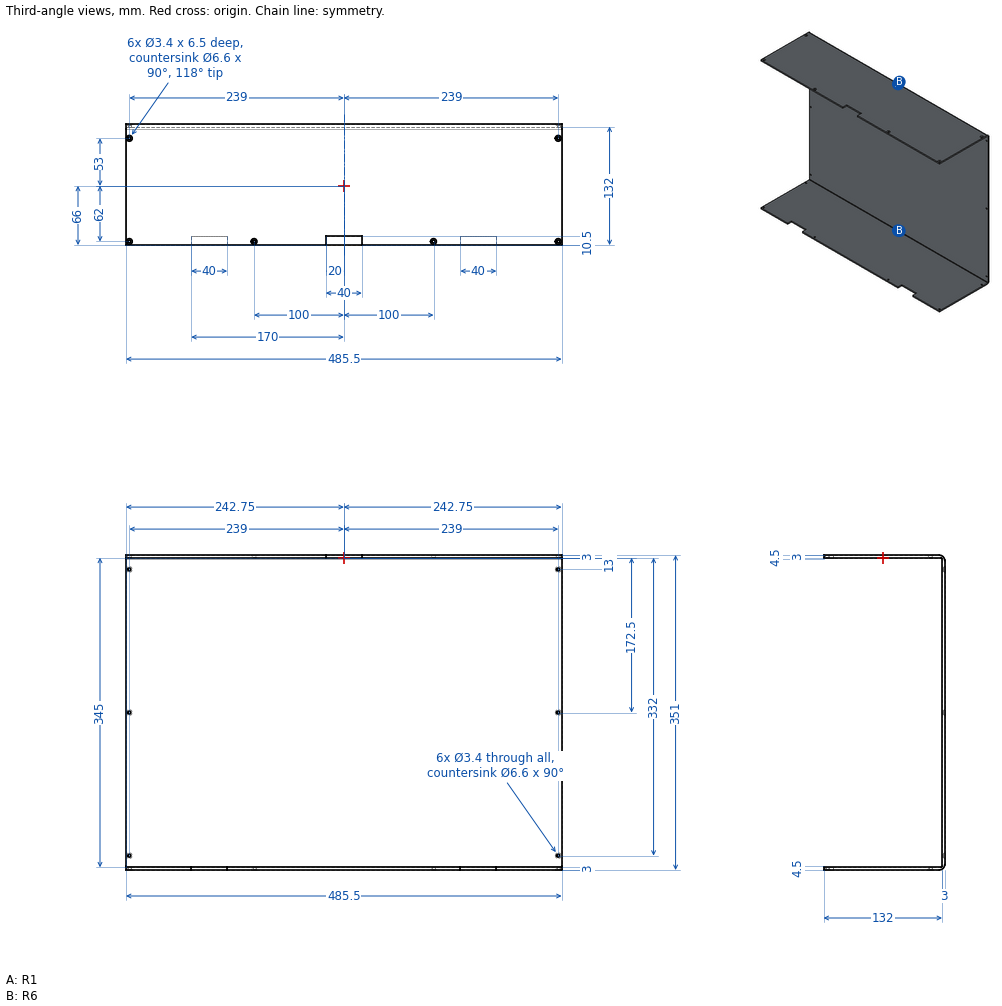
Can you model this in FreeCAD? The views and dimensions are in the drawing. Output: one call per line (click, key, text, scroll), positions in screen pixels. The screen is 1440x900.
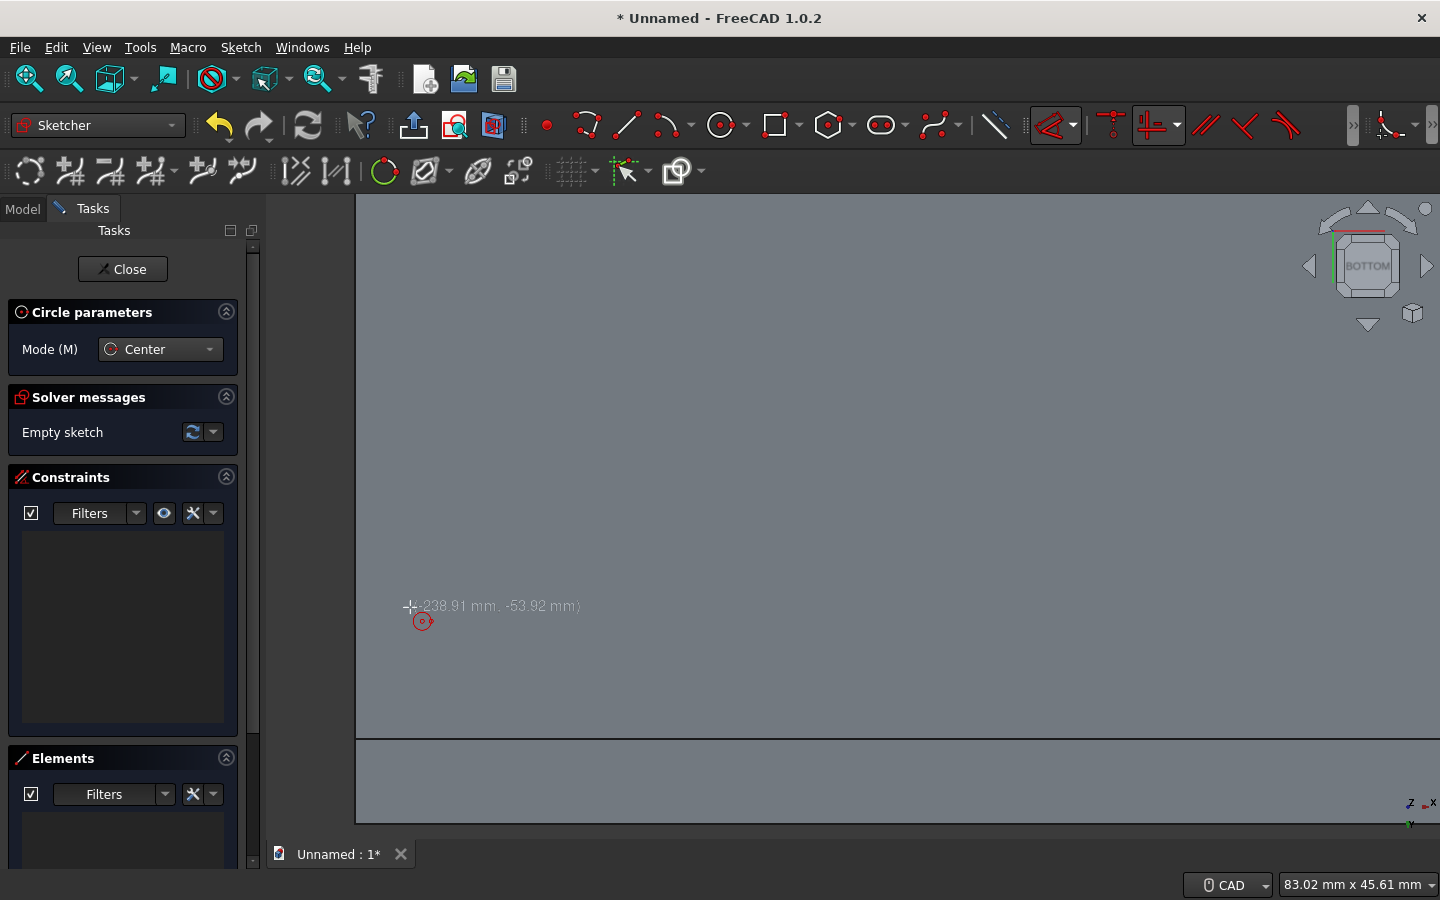
scroll(410, 608, down, 11)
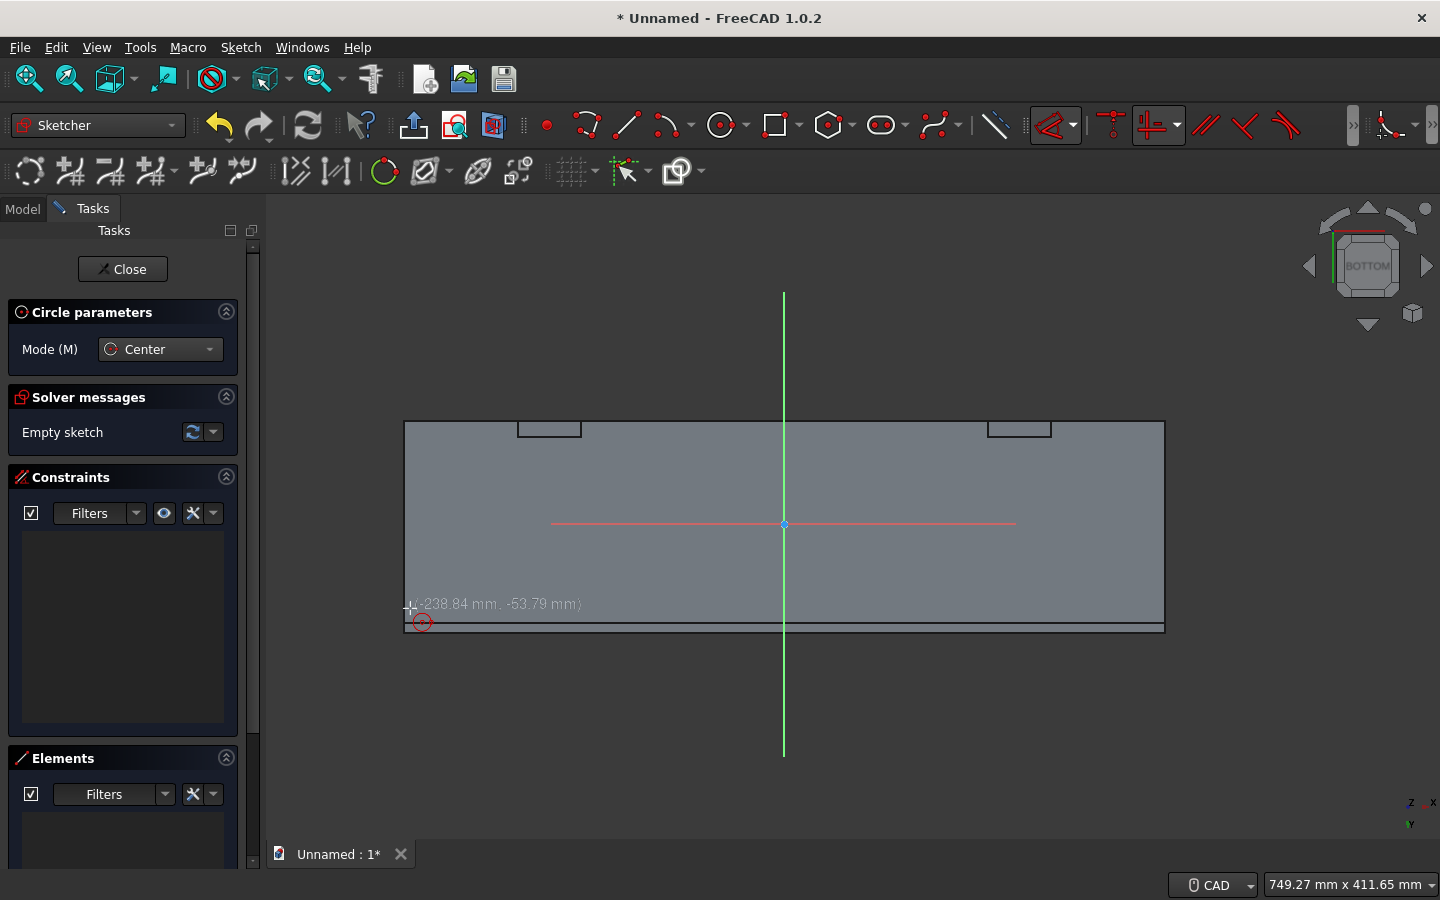
click(410, 607)
move(412, 606)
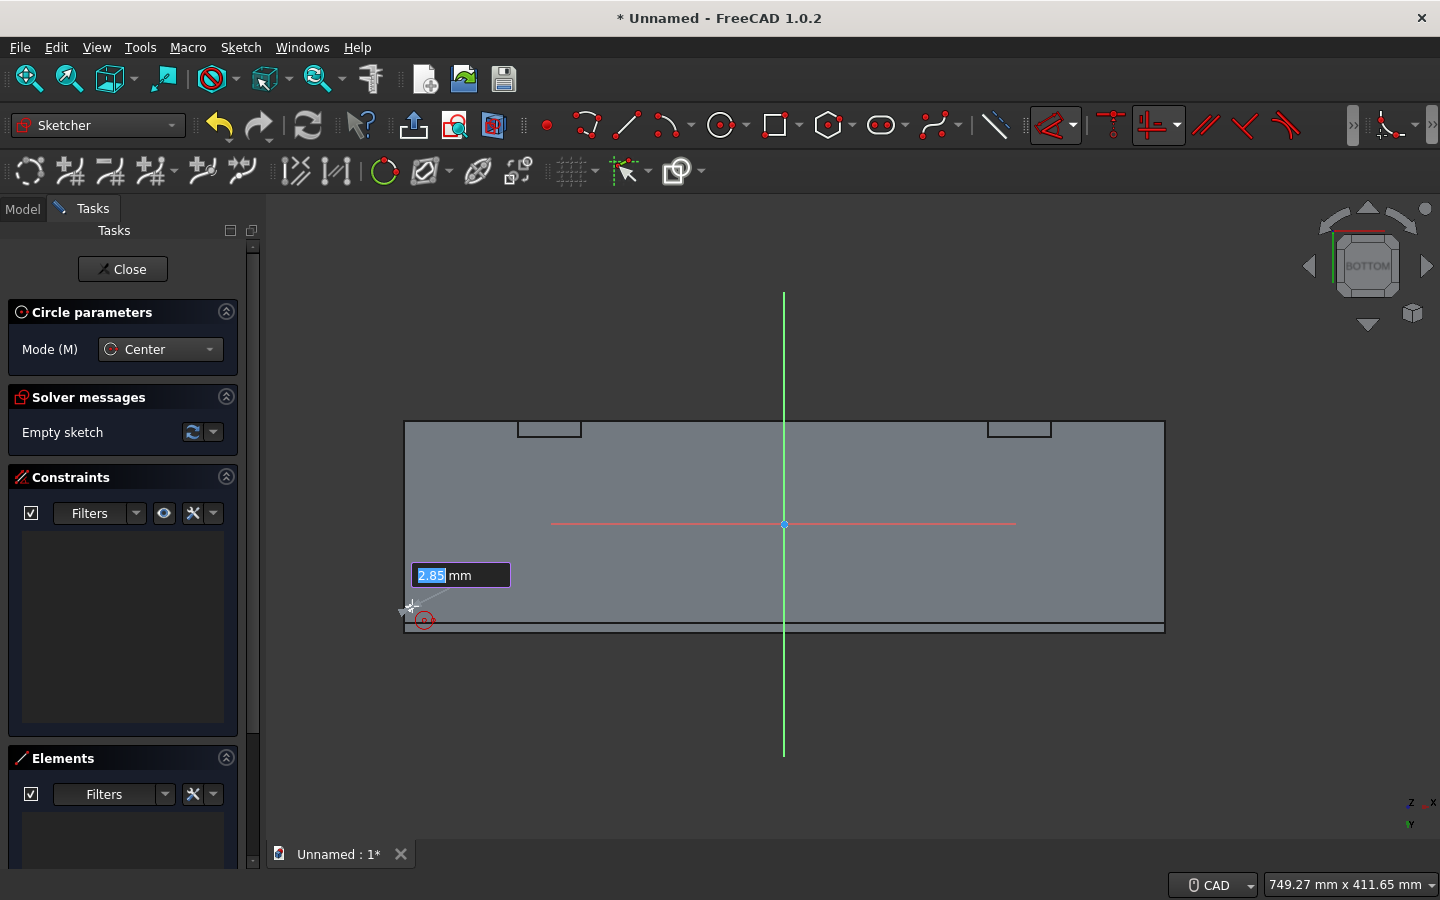
text(3.4)
key(Return)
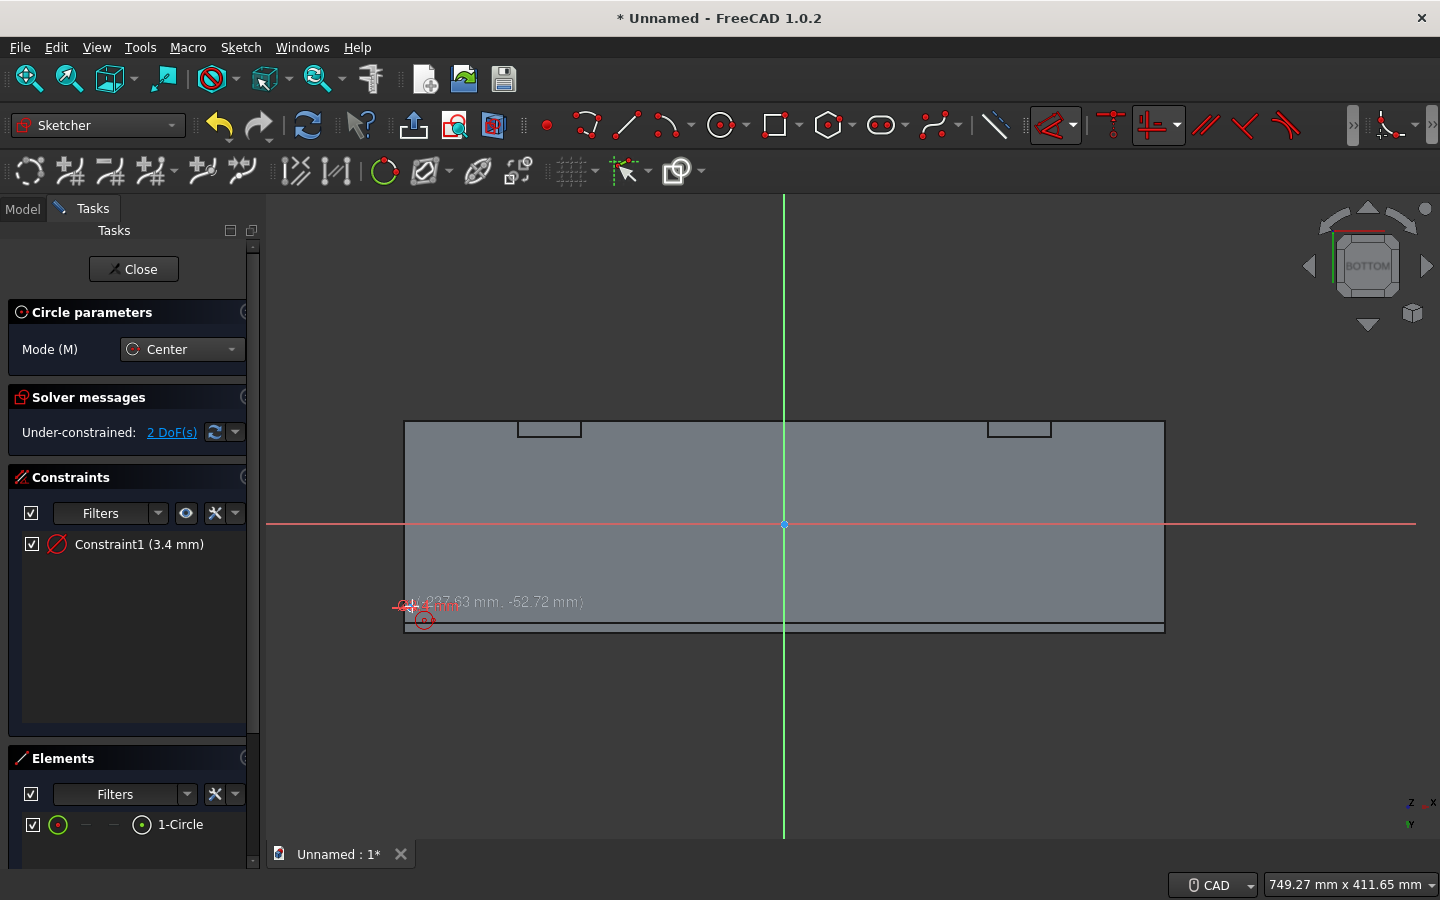
scroll(410, 427, up, 11)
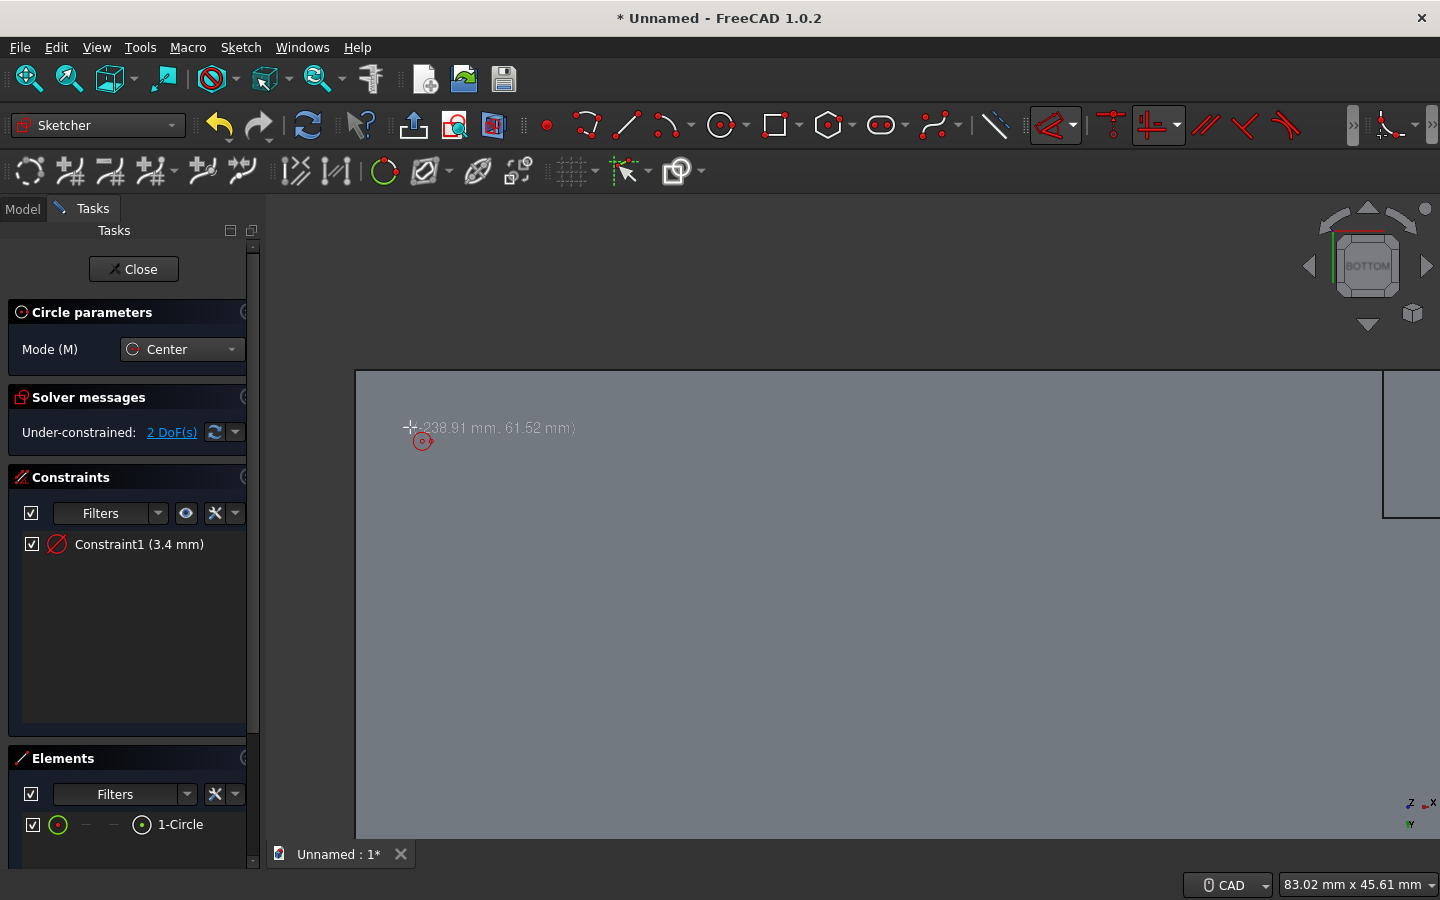
scroll(410, 426, down, 11)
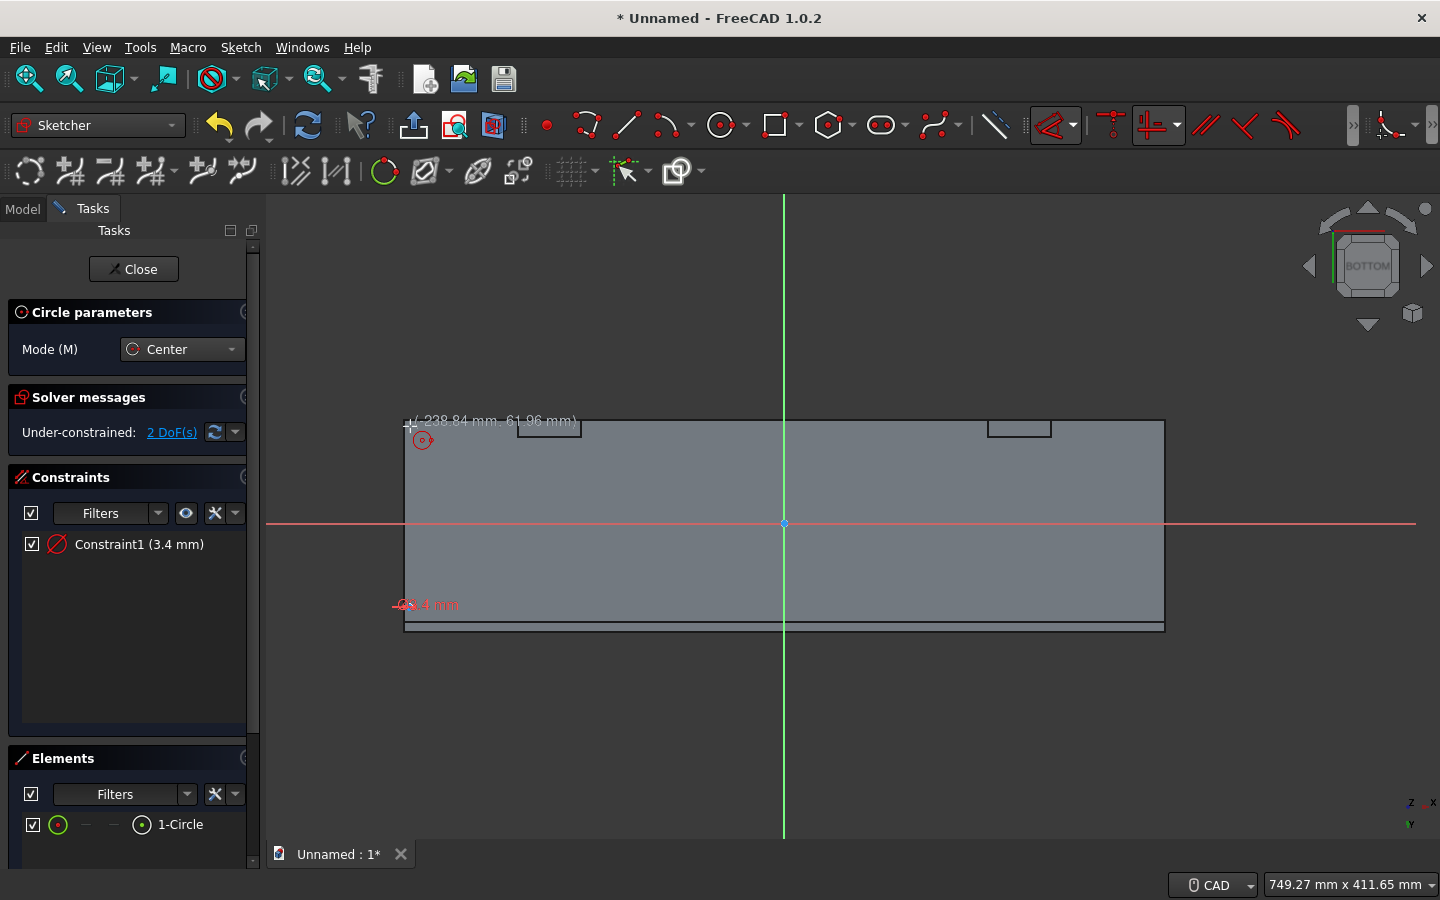
click(410, 426)
move(412, 424)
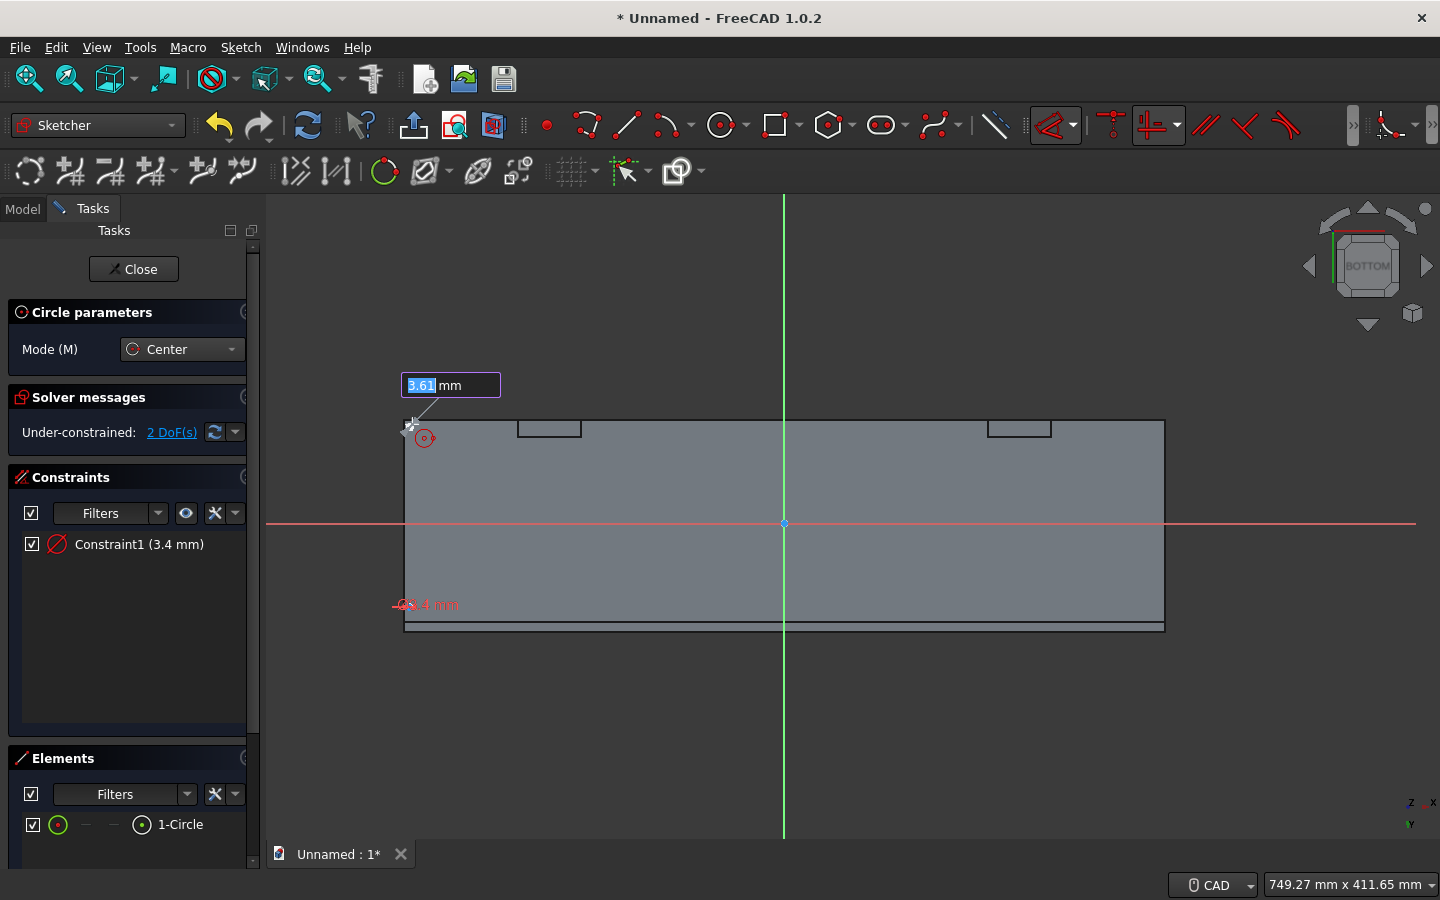
text(3.4)
key(Return)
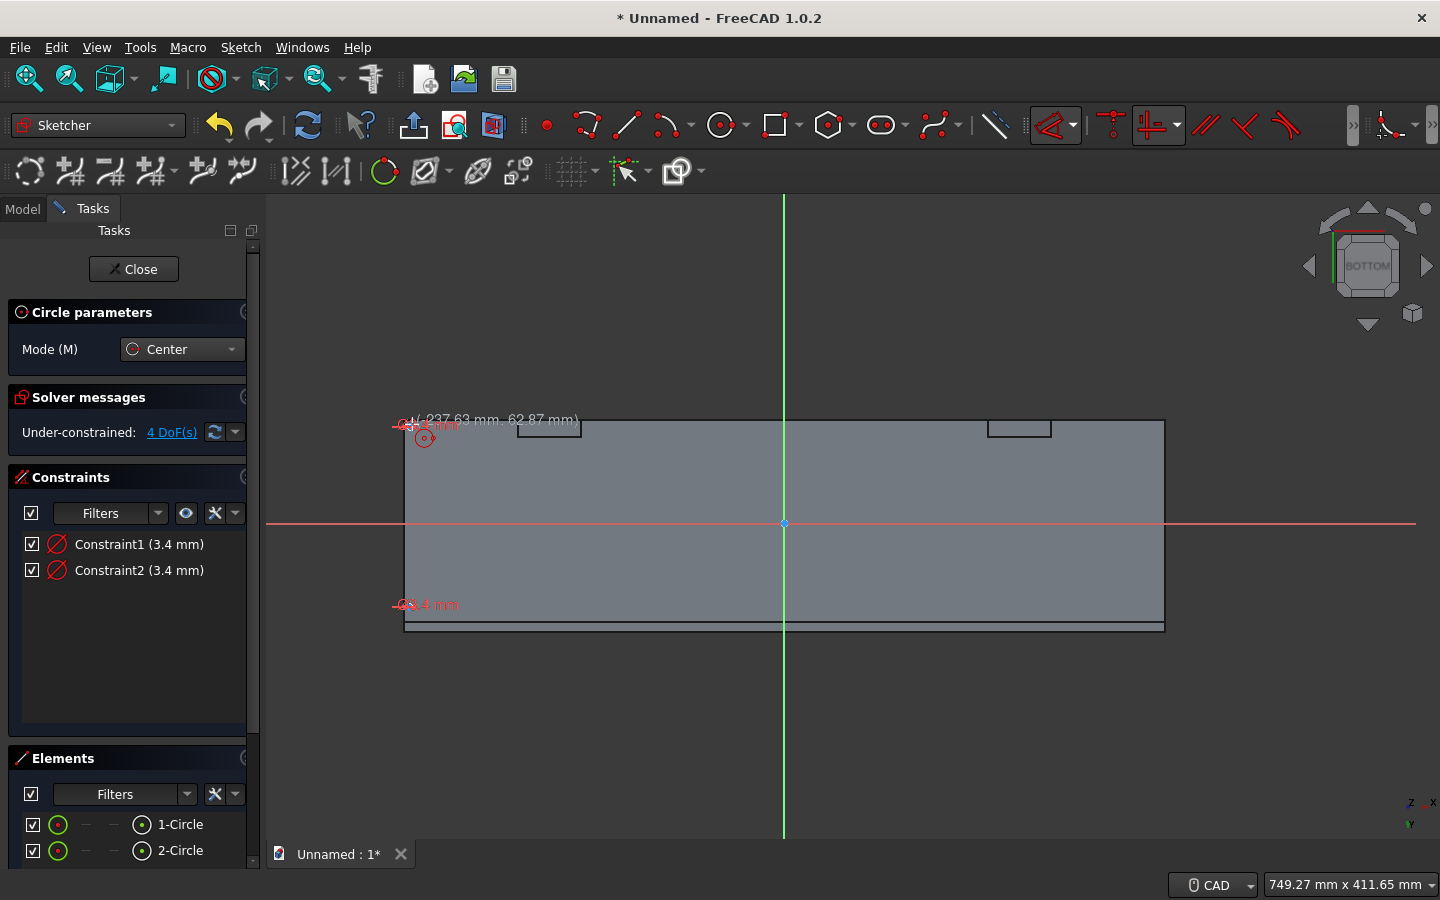
scroll(628, 426, up, 11)